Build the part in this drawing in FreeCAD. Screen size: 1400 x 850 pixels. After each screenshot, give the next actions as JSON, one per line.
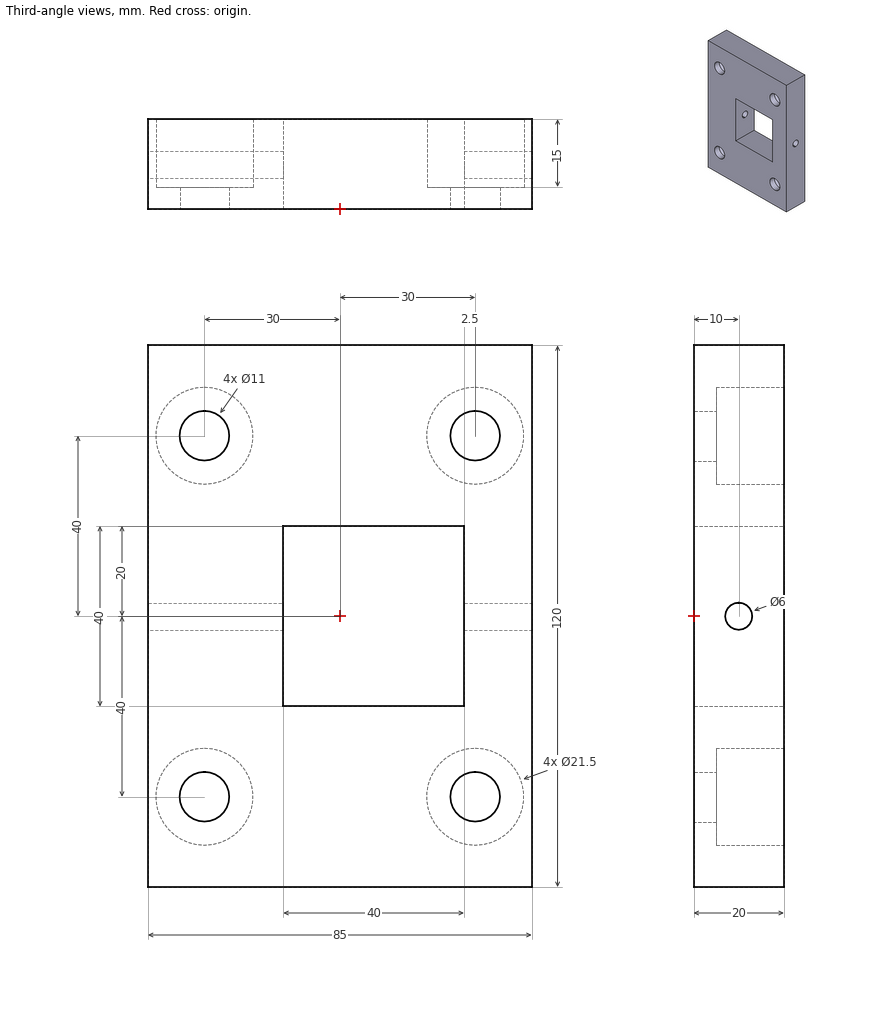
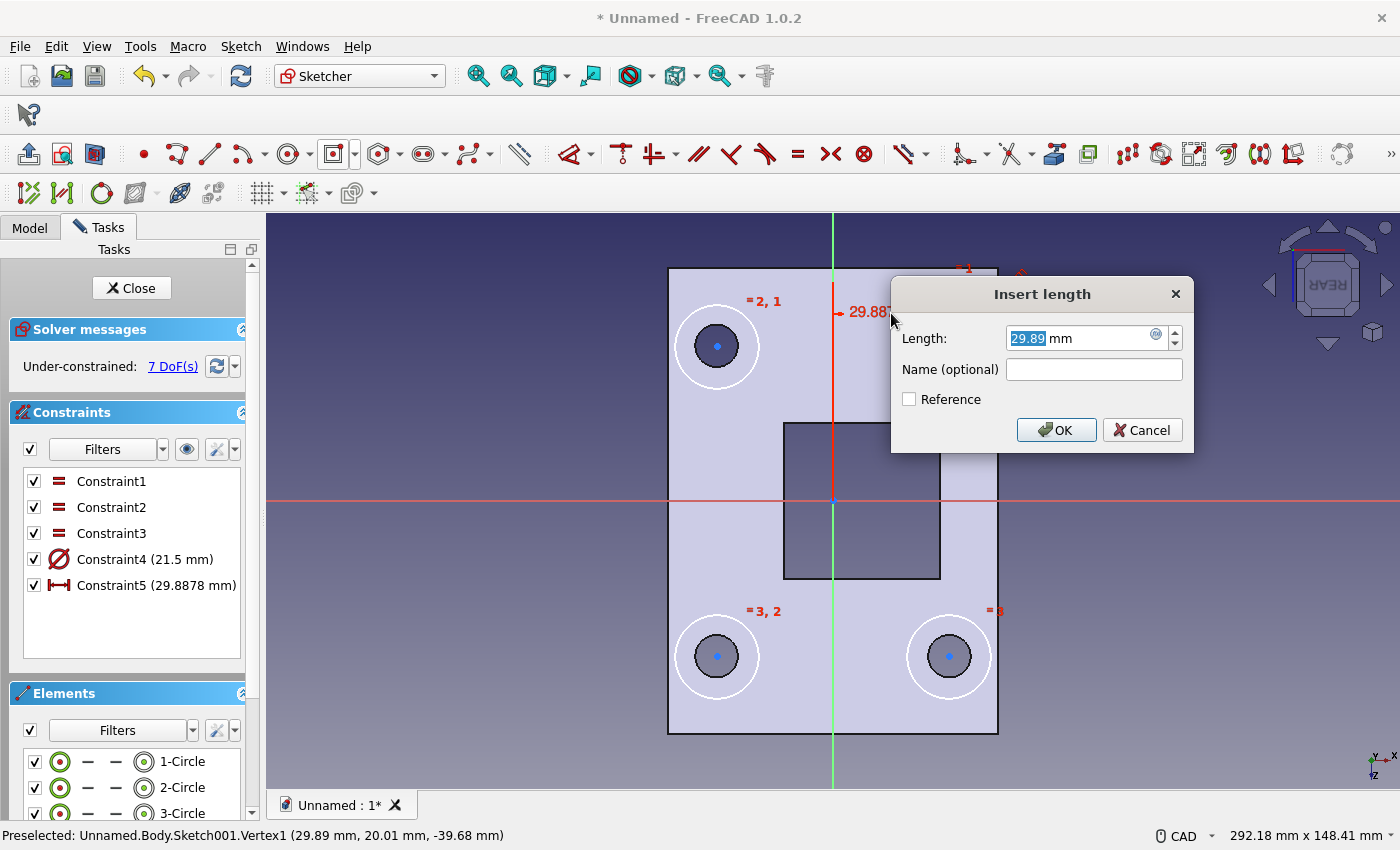
{"action": "type", "text": "30"}
{"action": "key", "text": "Return"}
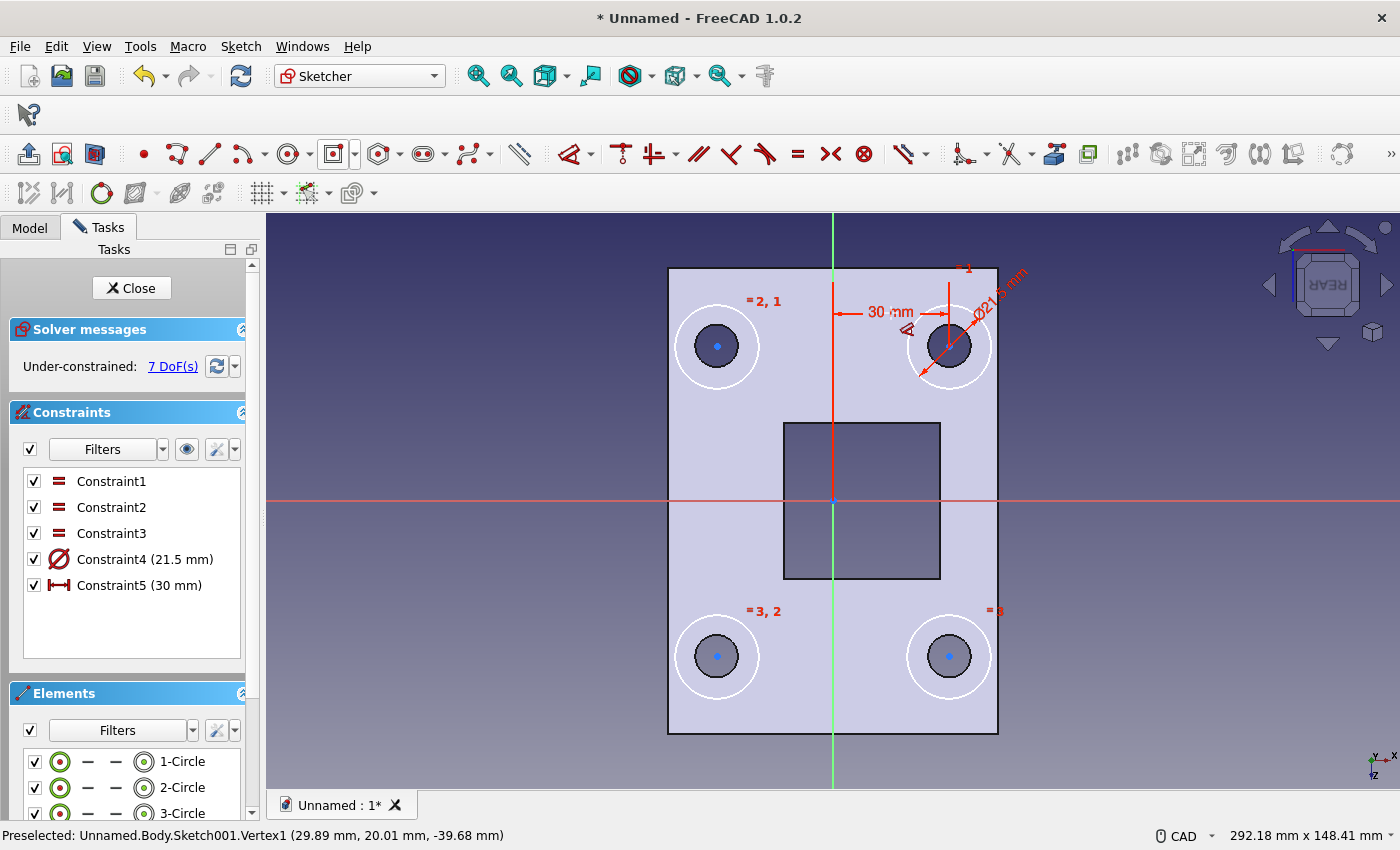
{"action": "left_click", "coordinate": [949, 347]}
{"action": "left_click", "coordinate": [983, 424]}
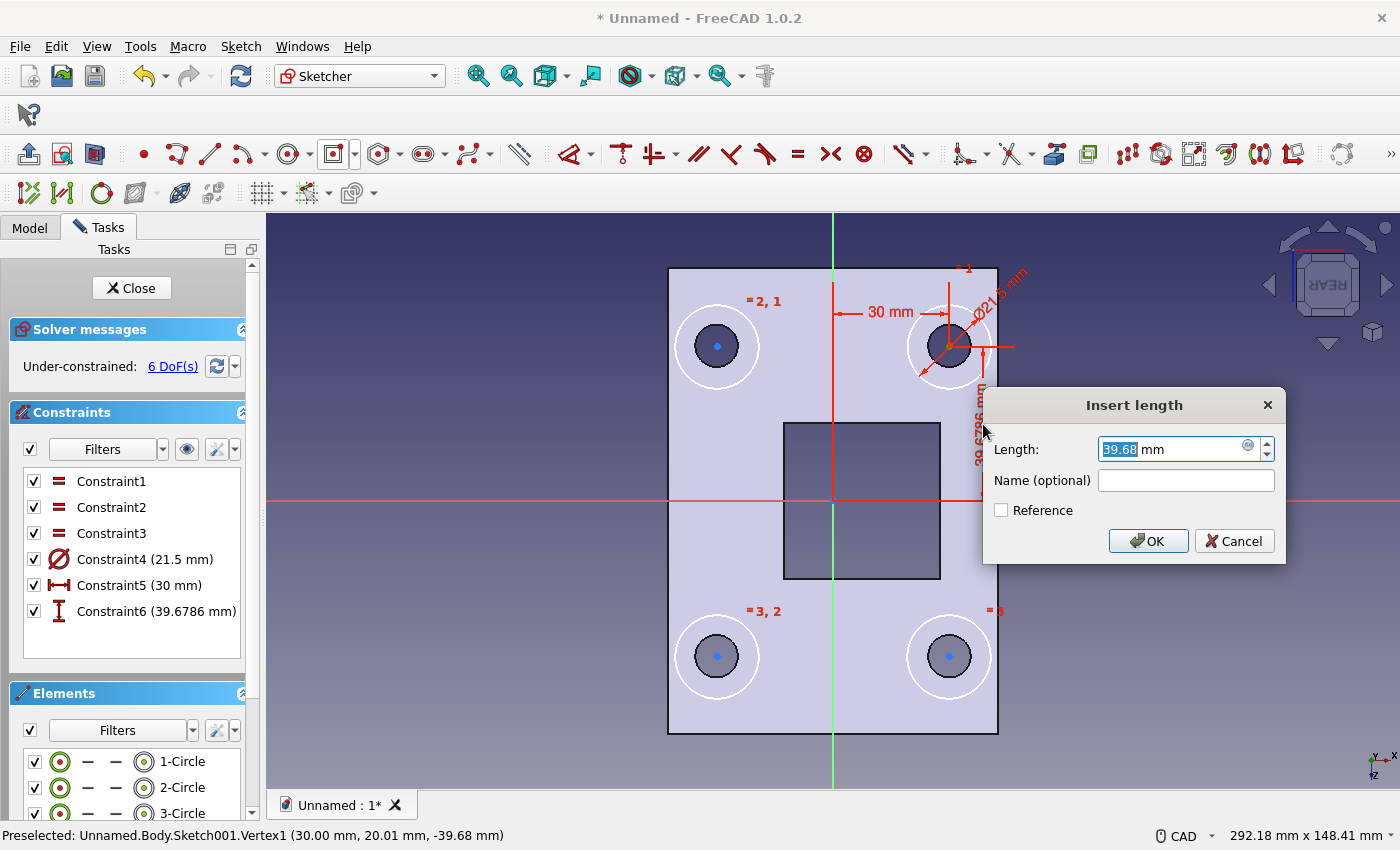
{"action": "type", "text": "40"}
{"action": "key", "text": "Return"}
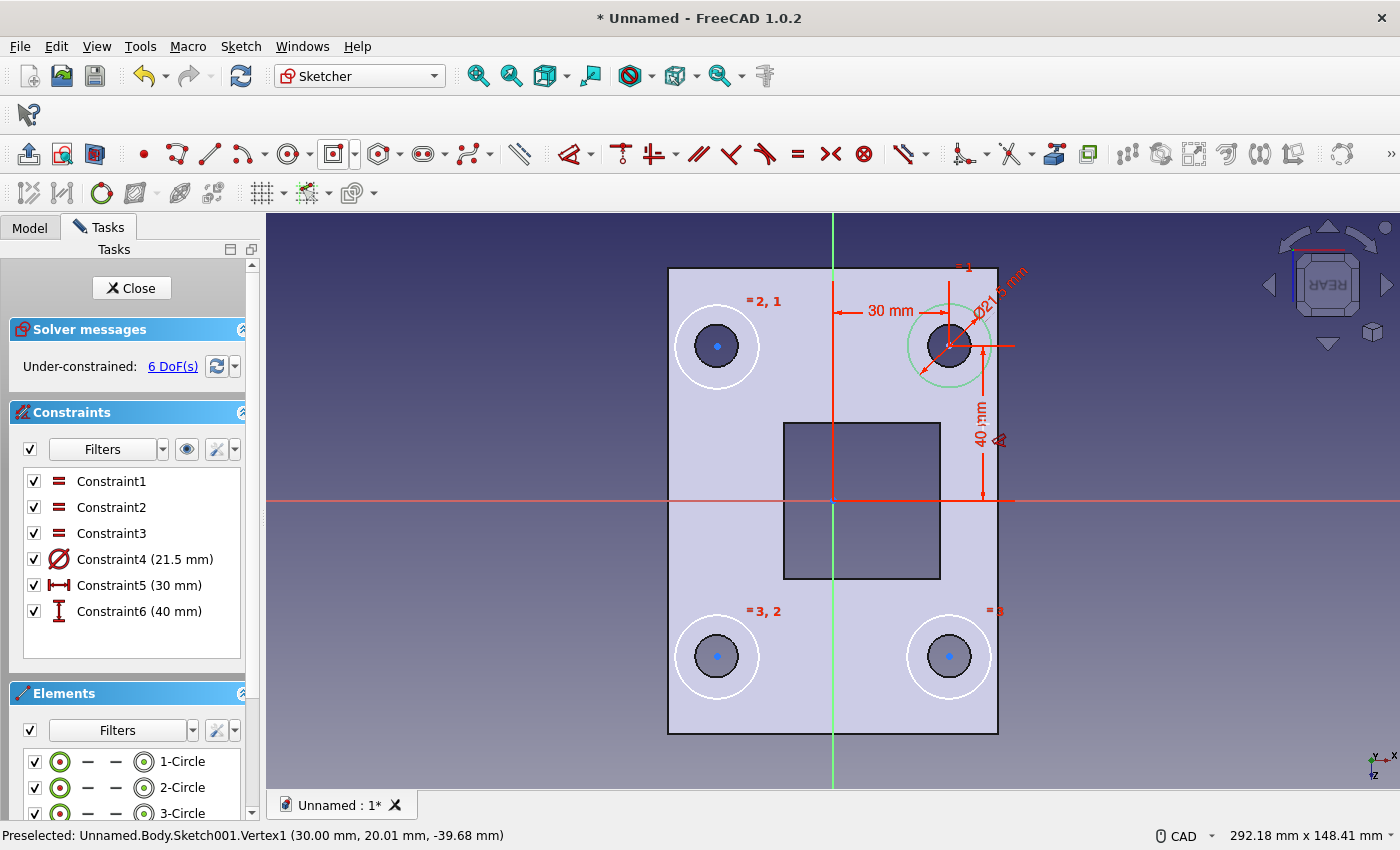
{"action": "left_click", "coordinate": [717, 347]}
{"action": "left_click", "coordinate": [775, 313]}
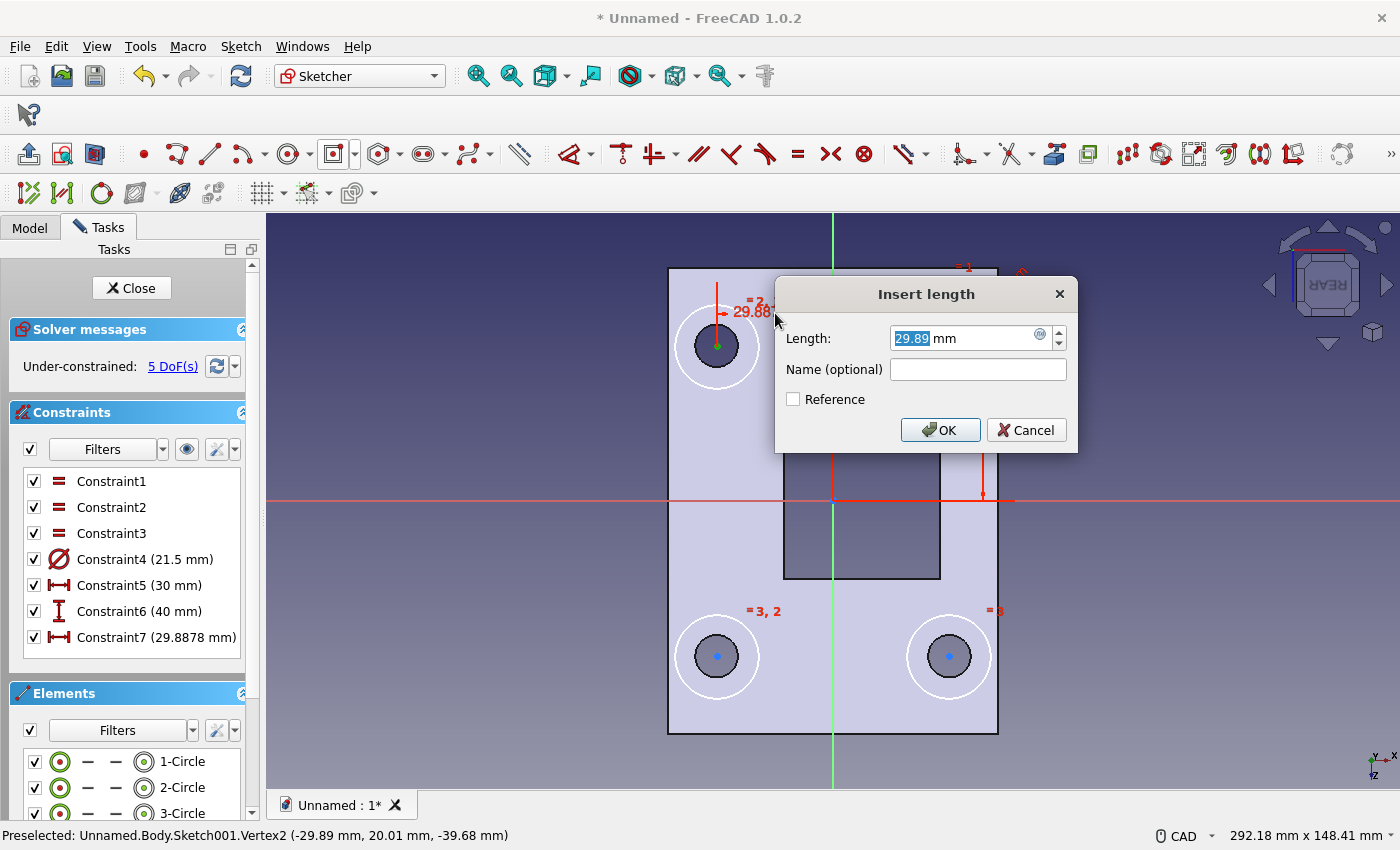
{"action": "type", "text": "30"}
{"action": "key", "text": "Return"}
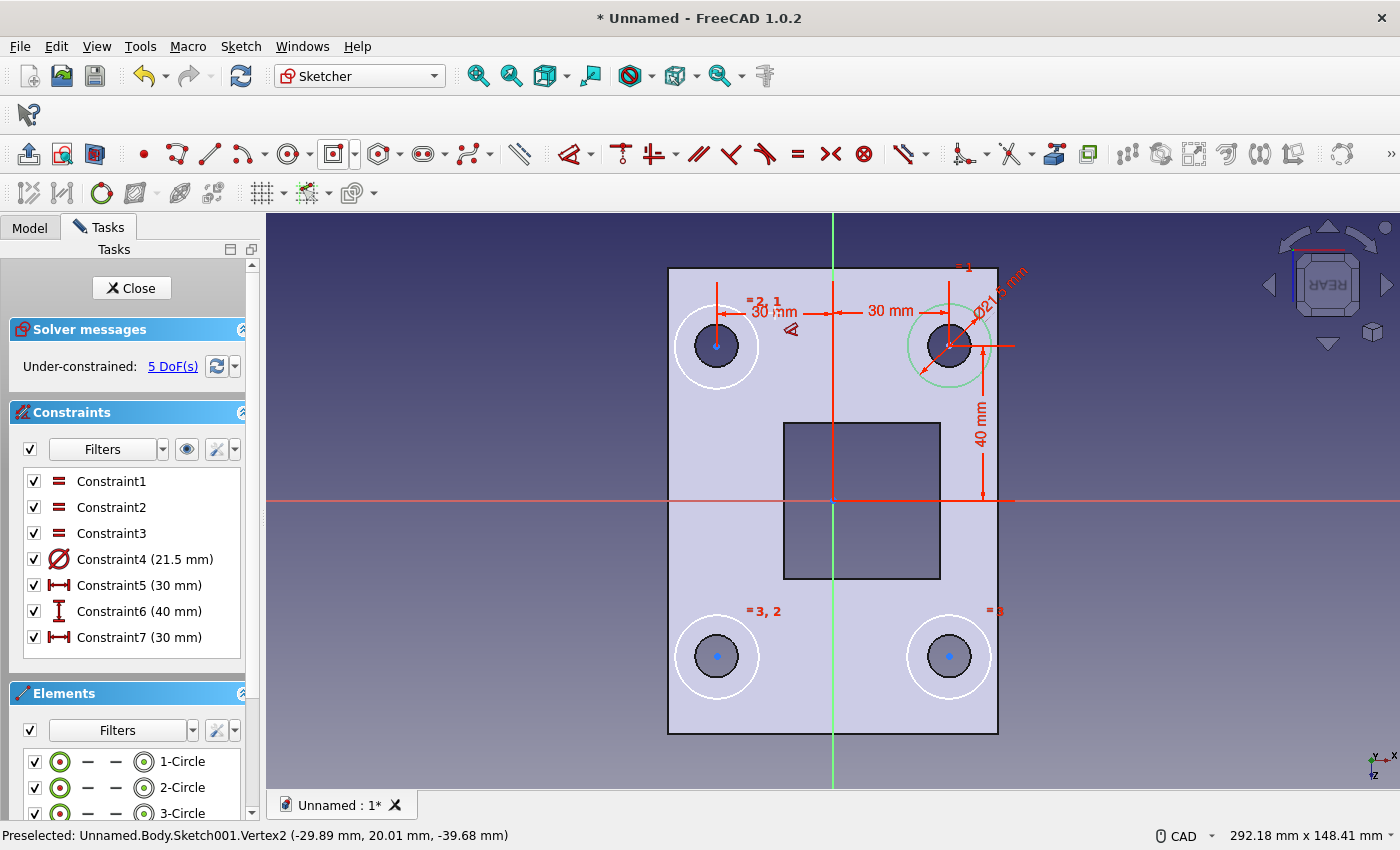
{"action": "left_click", "coordinate": [717, 347]}
{"action": "left_click", "coordinate": [683, 424]}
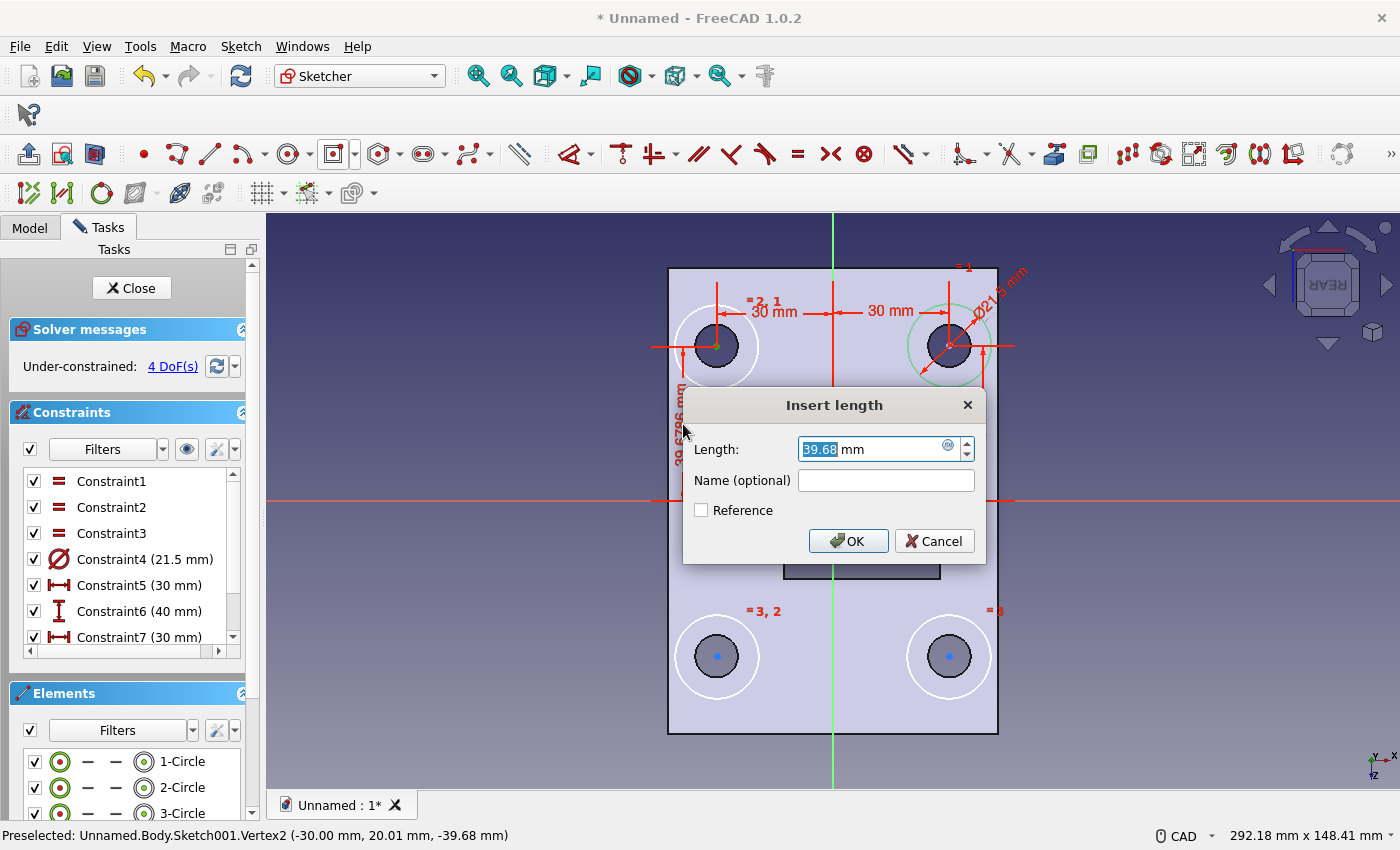
{"action": "type", "text": "40"}
{"action": "key", "text": "Return"}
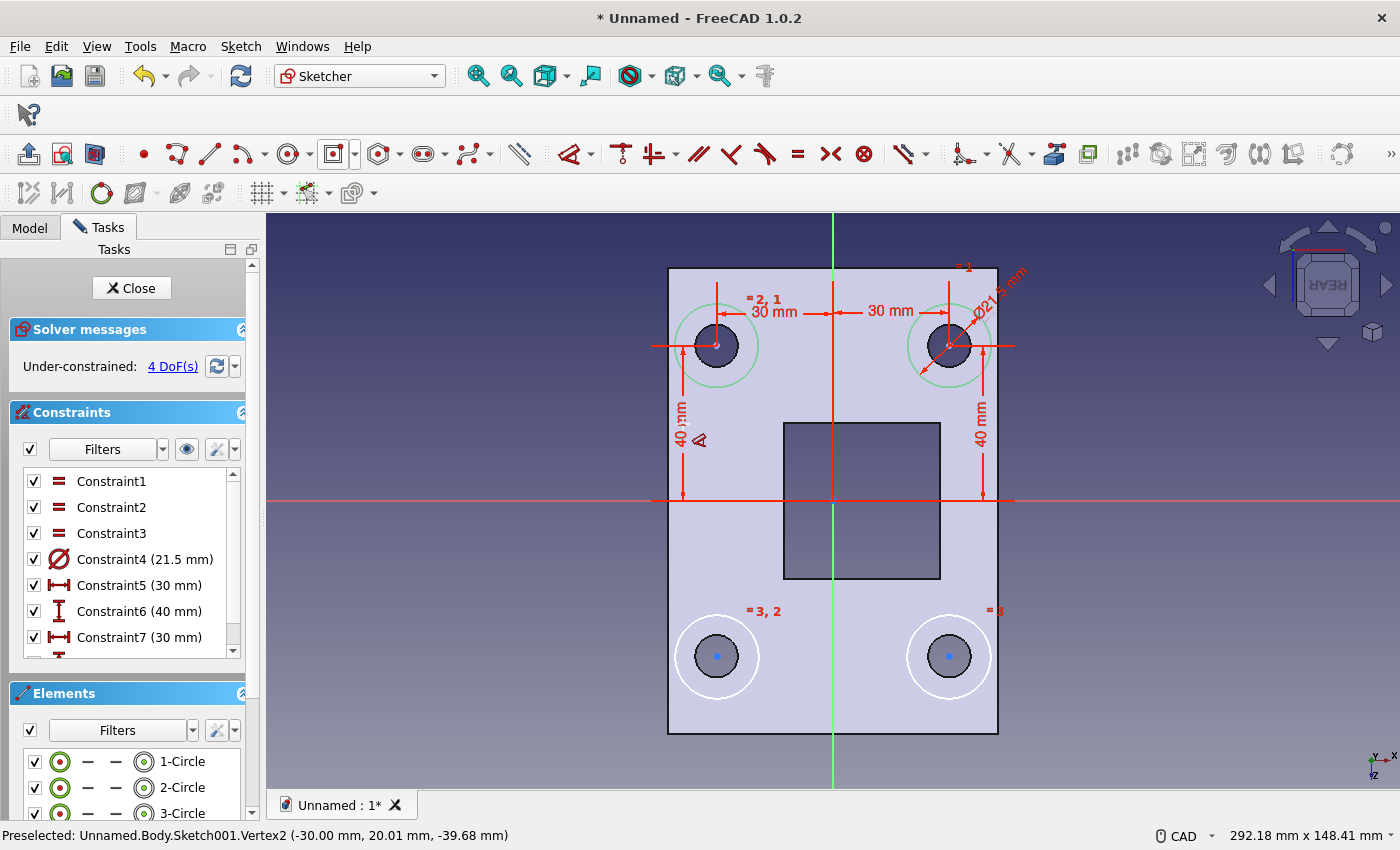
{"action": "left_click", "coordinate": [717, 657]}
{"action": "left_click", "coordinate": [775, 691]}